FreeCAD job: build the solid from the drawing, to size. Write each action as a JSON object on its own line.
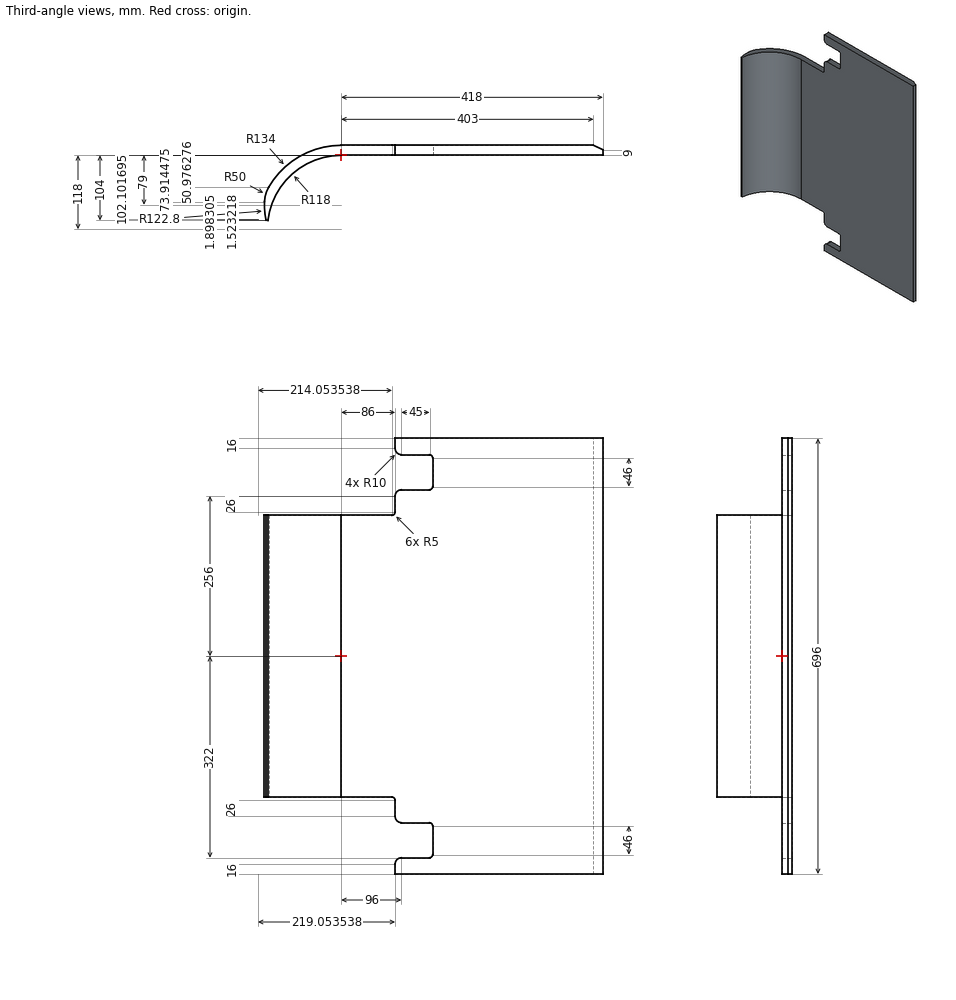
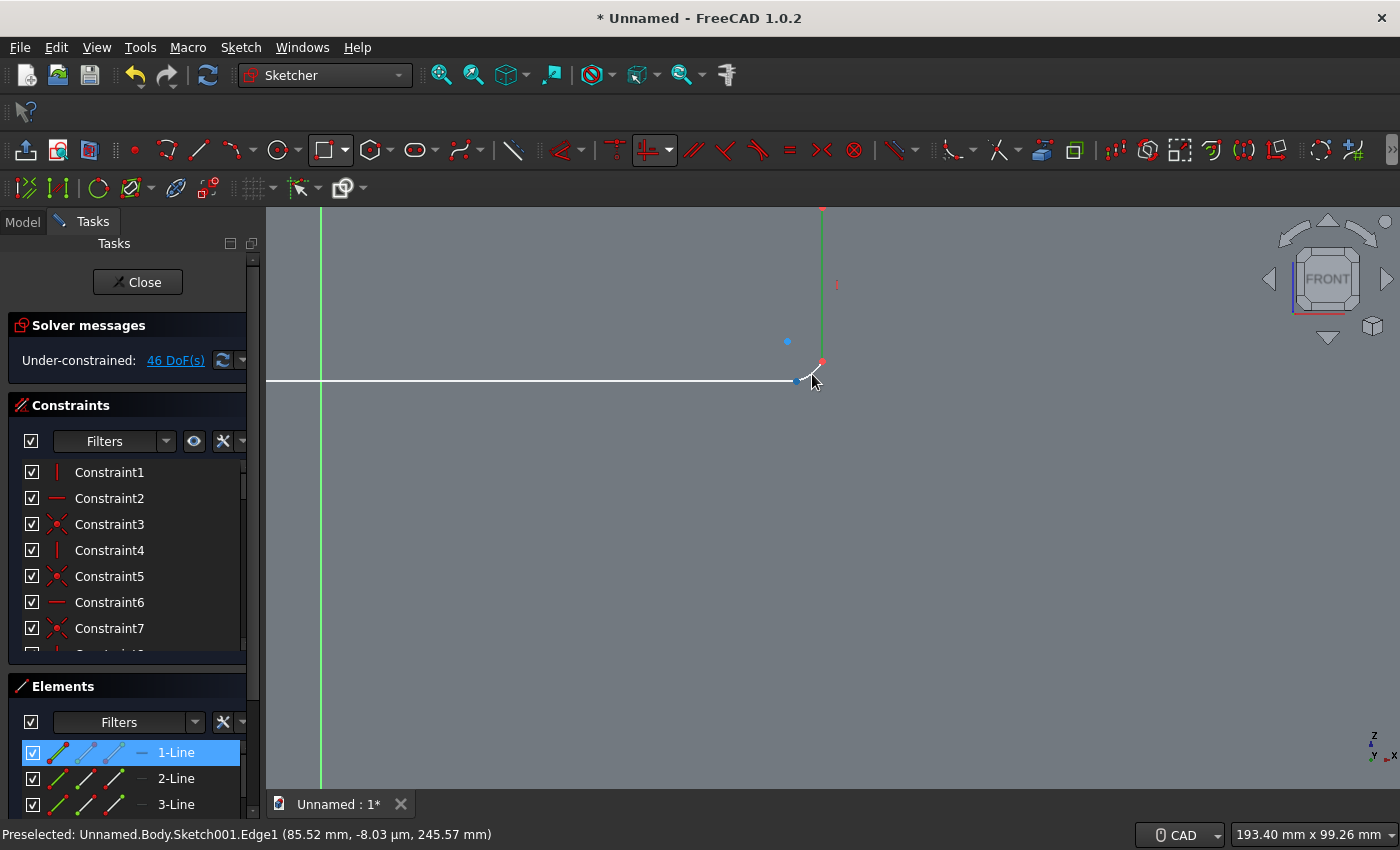
{"action": "left_click", "coordinate": [811, 374]}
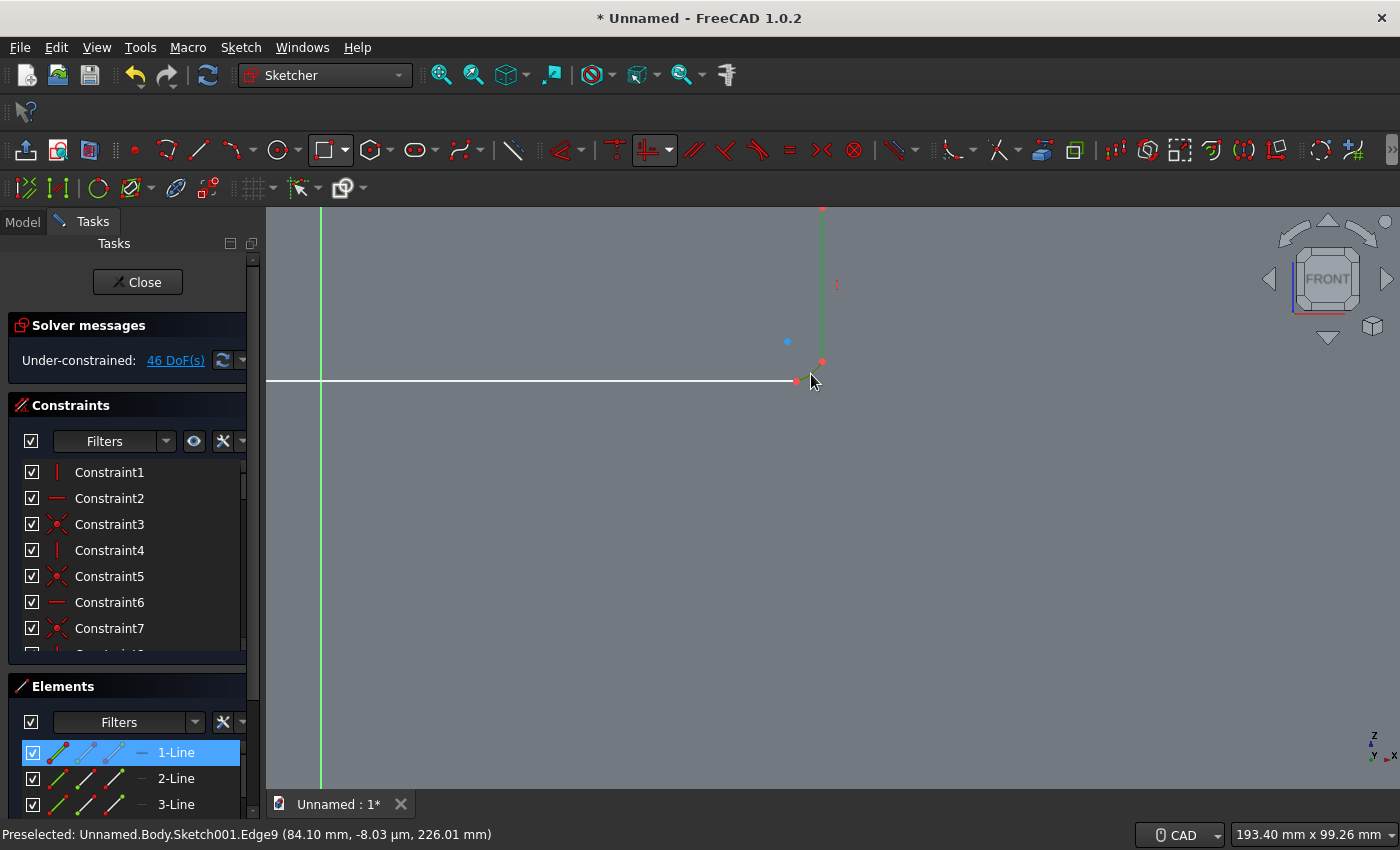
{"action": "left_click", "coordinate": [758, 150]}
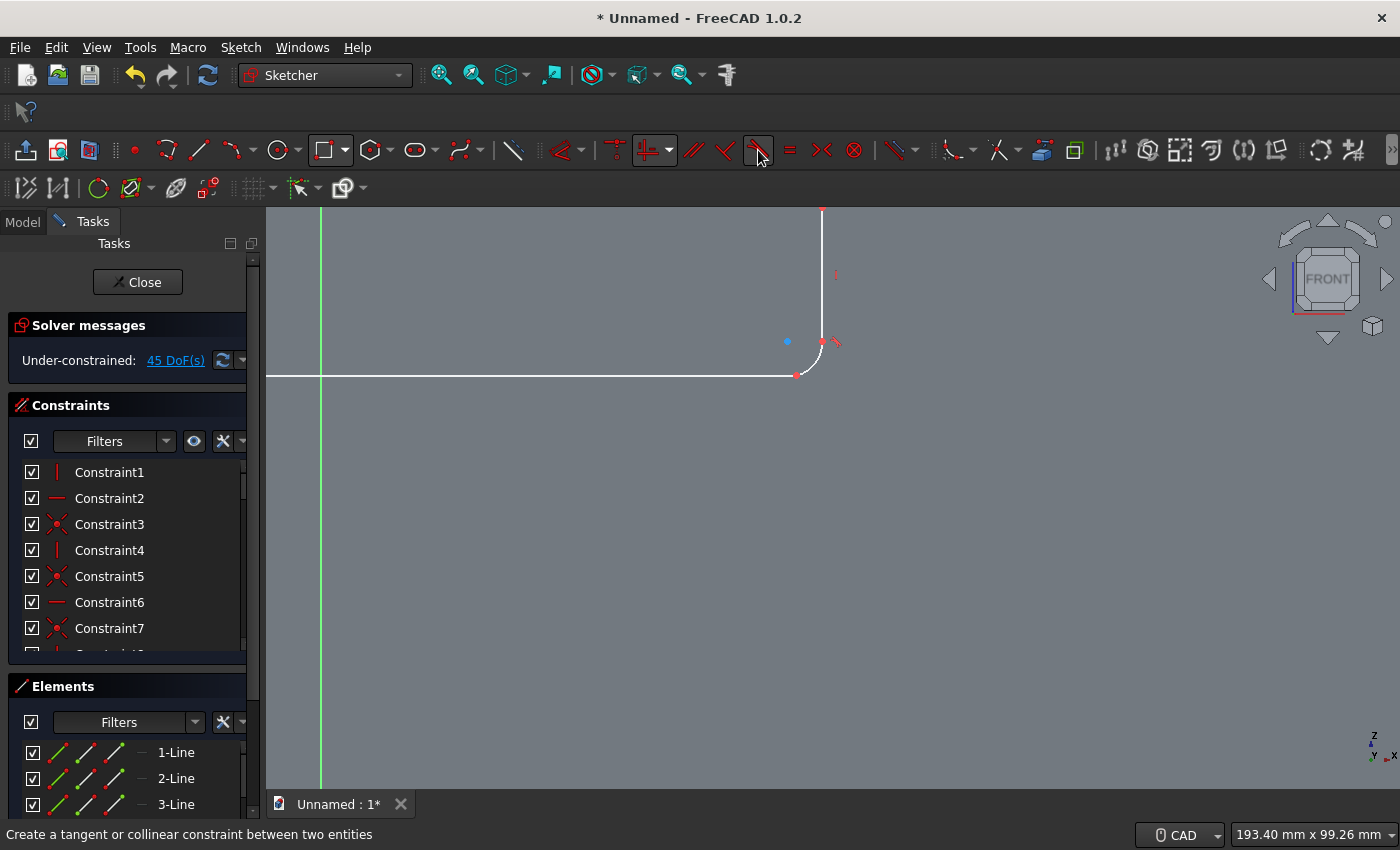
{"action": "scroll", "coordinate": [805, 378], "scroll_direction": "down", "scroll_amount": 12}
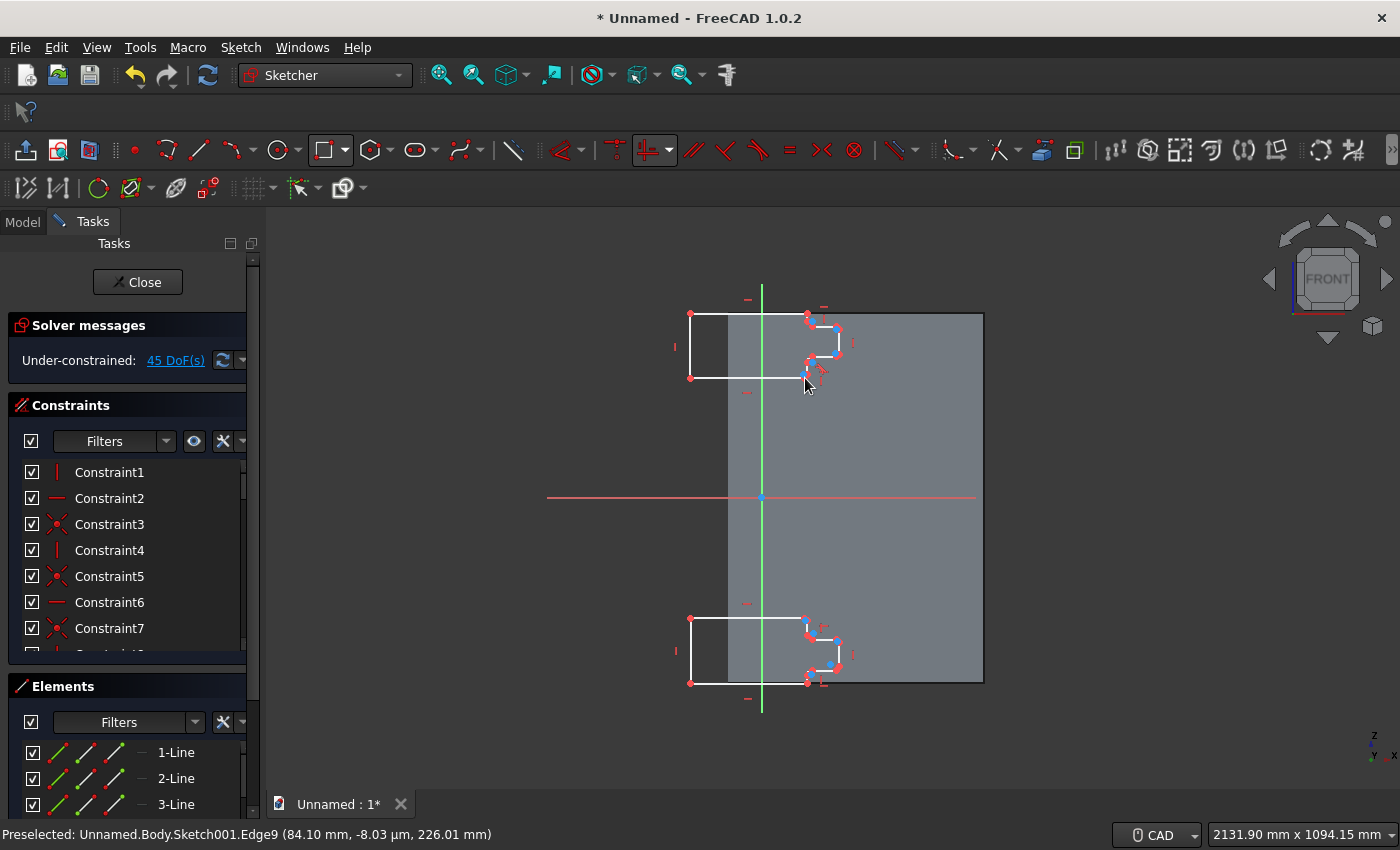
{"action": "scroll", "coordinate": [807, 366], "scroll_direction": "up", "scroll_amount": 7}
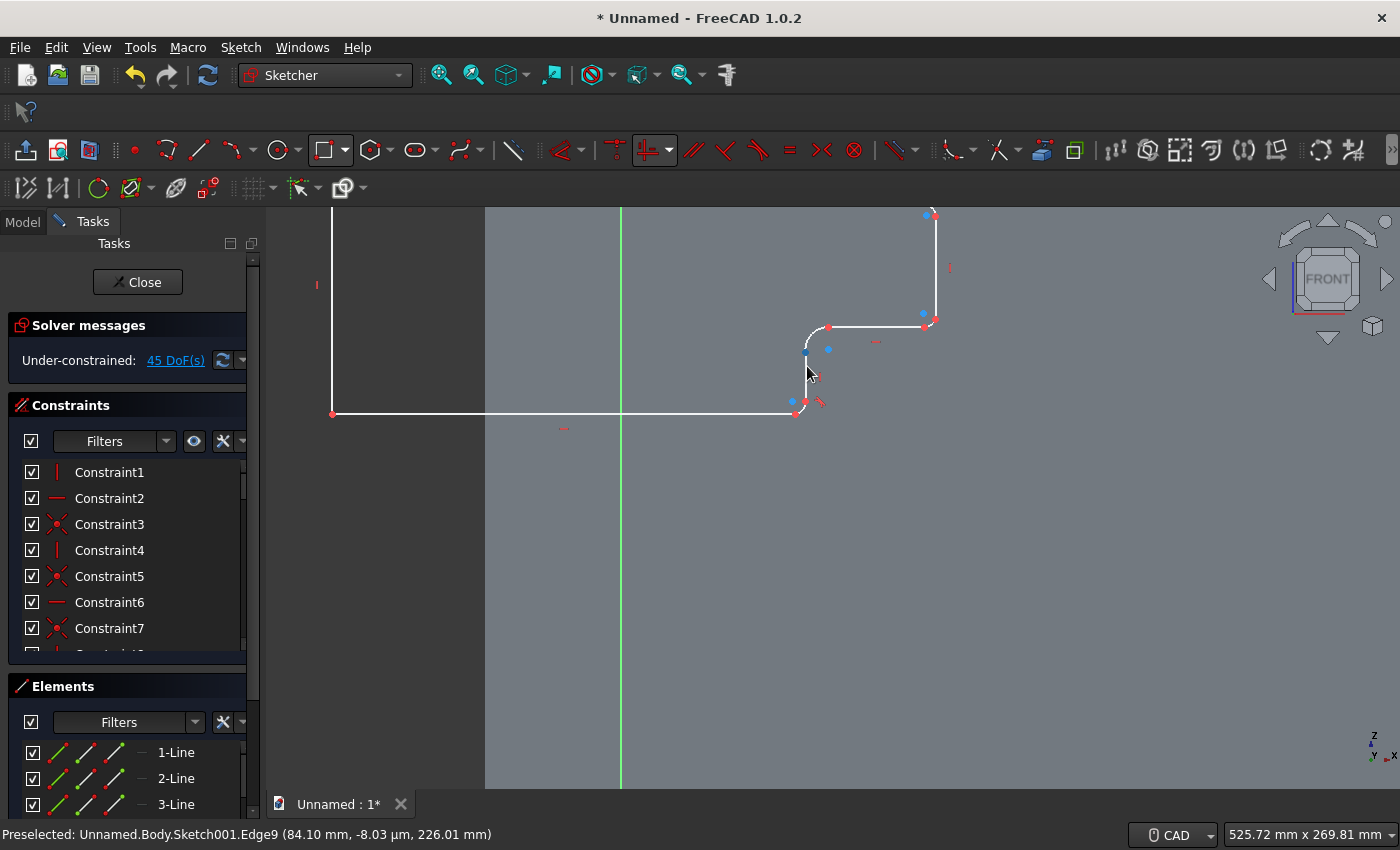
{"action": "left_click", "coordinate": [806, 367]}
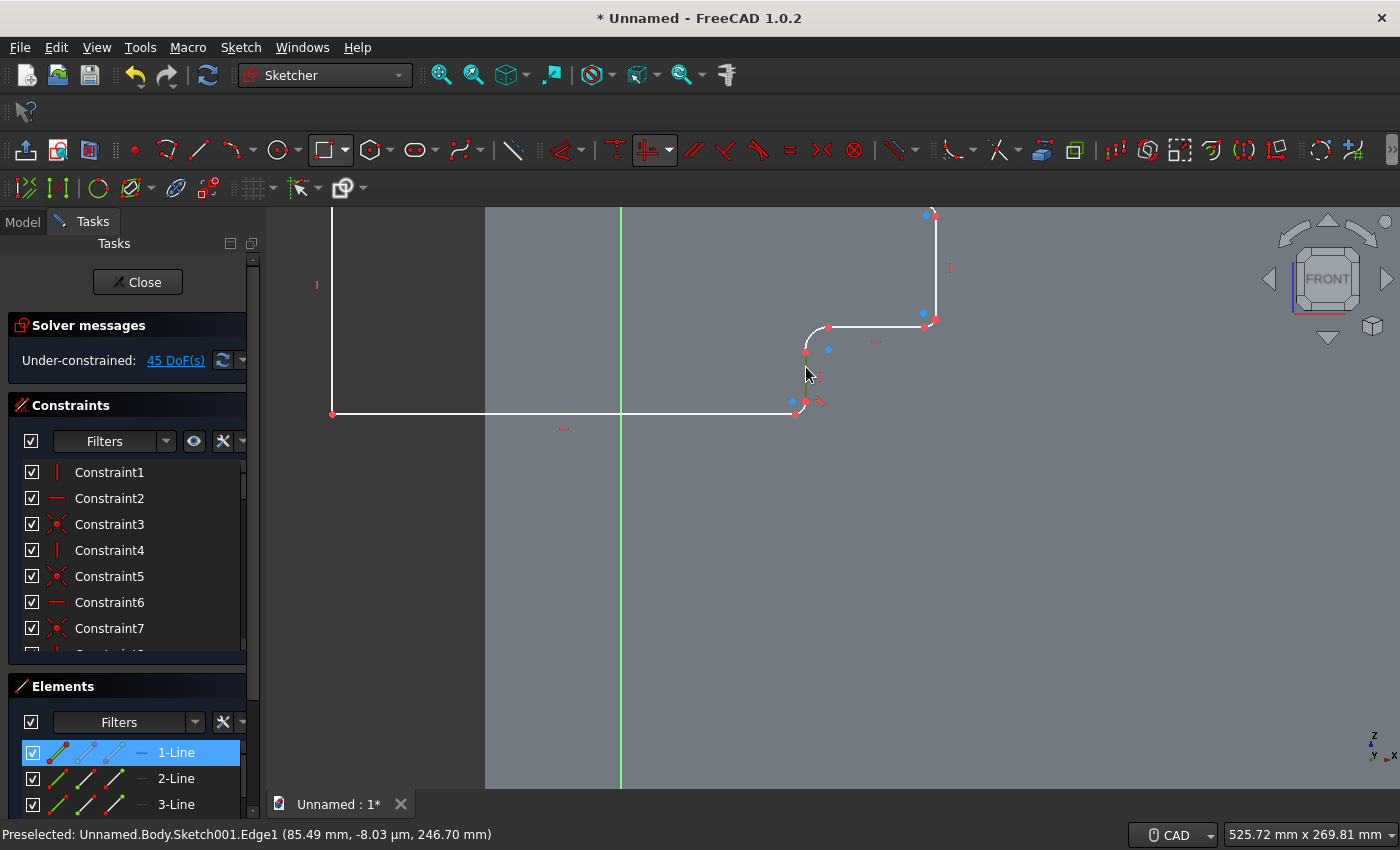
{"action": "left_click", "coordinate": [817, 330]}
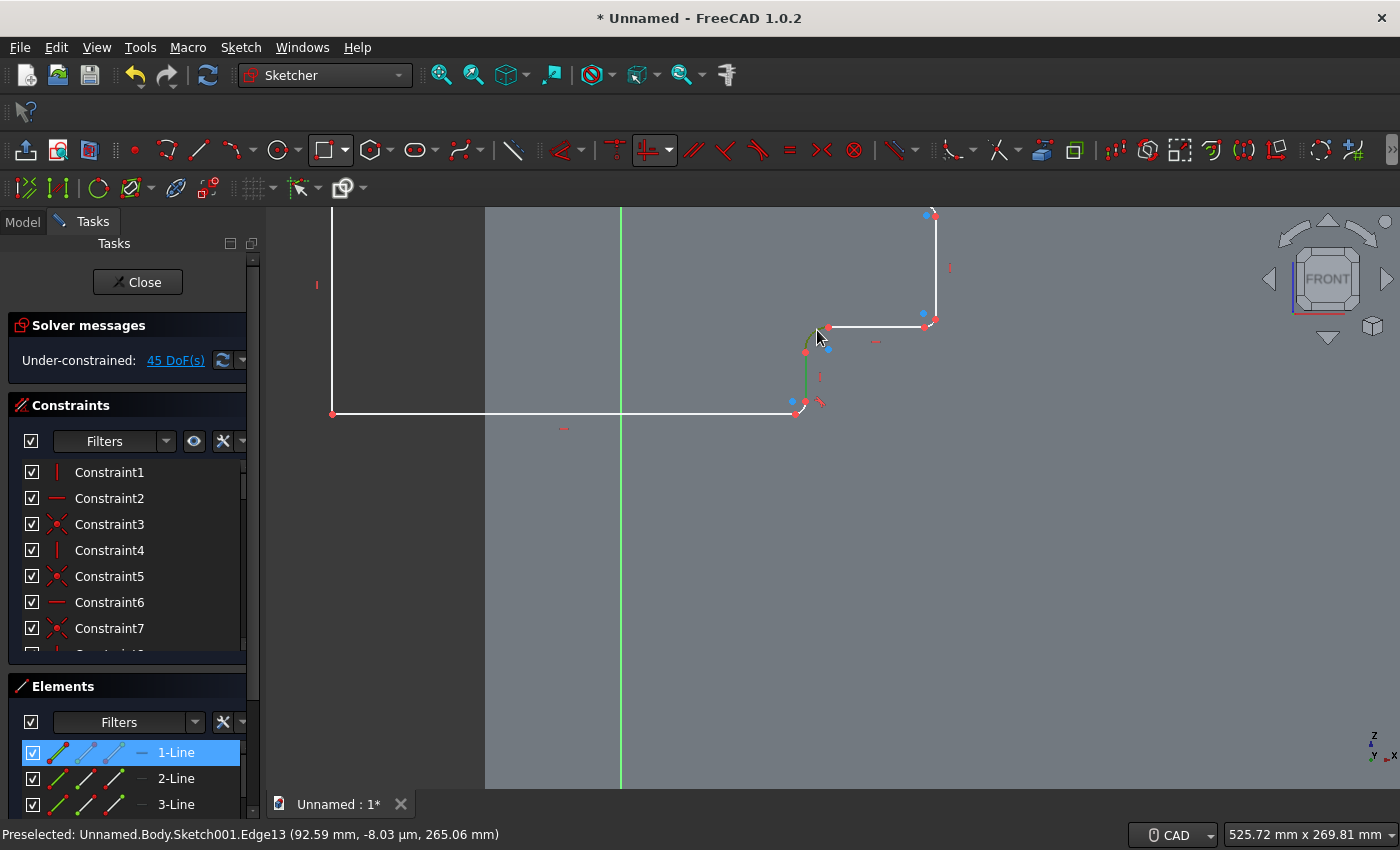
{"action": "left_click", "coordinate": [758, 150]}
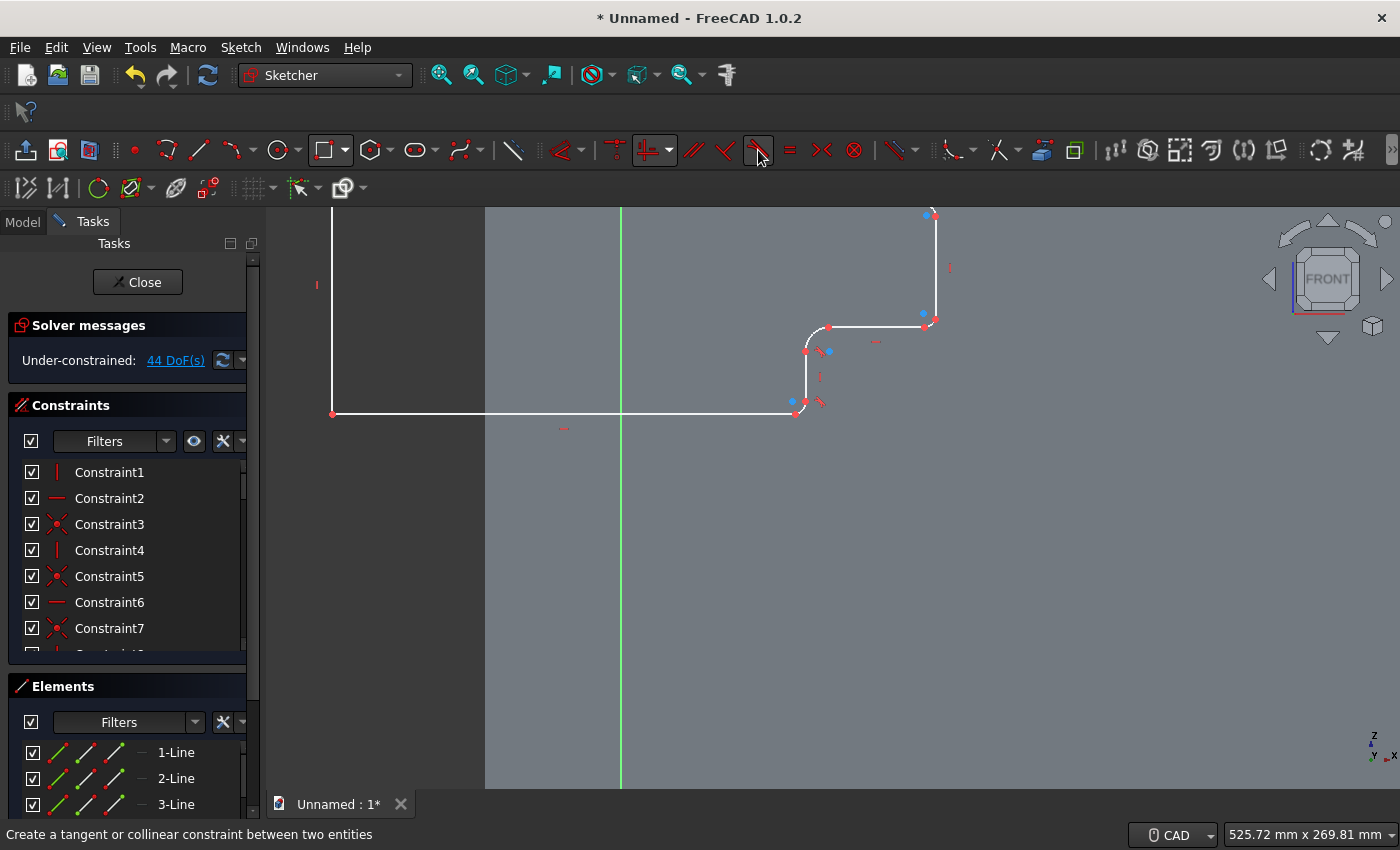
{"action": "left_click", "coordinate": [657, 414]}